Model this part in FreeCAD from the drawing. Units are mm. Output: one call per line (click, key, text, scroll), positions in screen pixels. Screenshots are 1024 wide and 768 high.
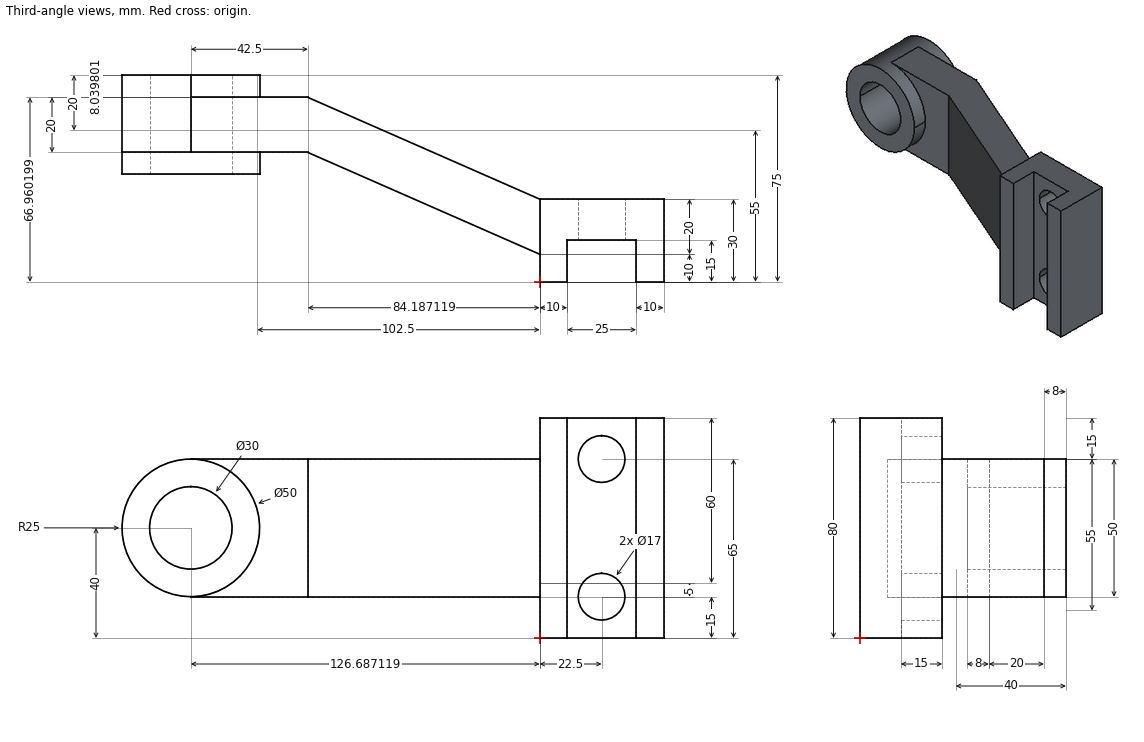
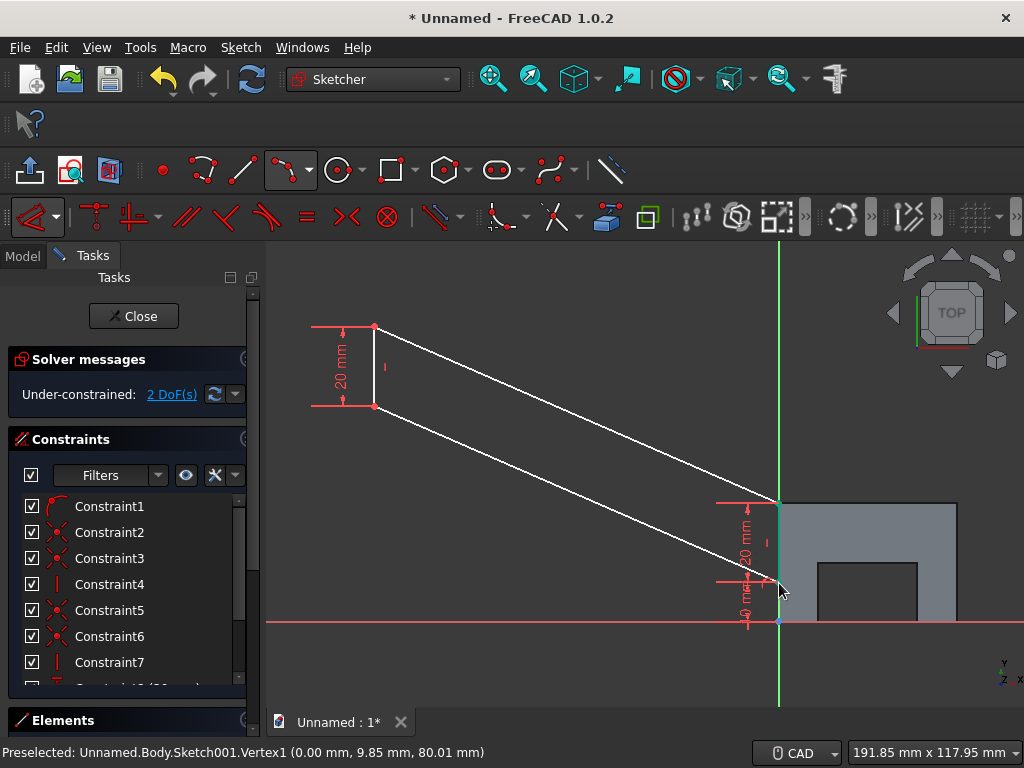
click(374, 327)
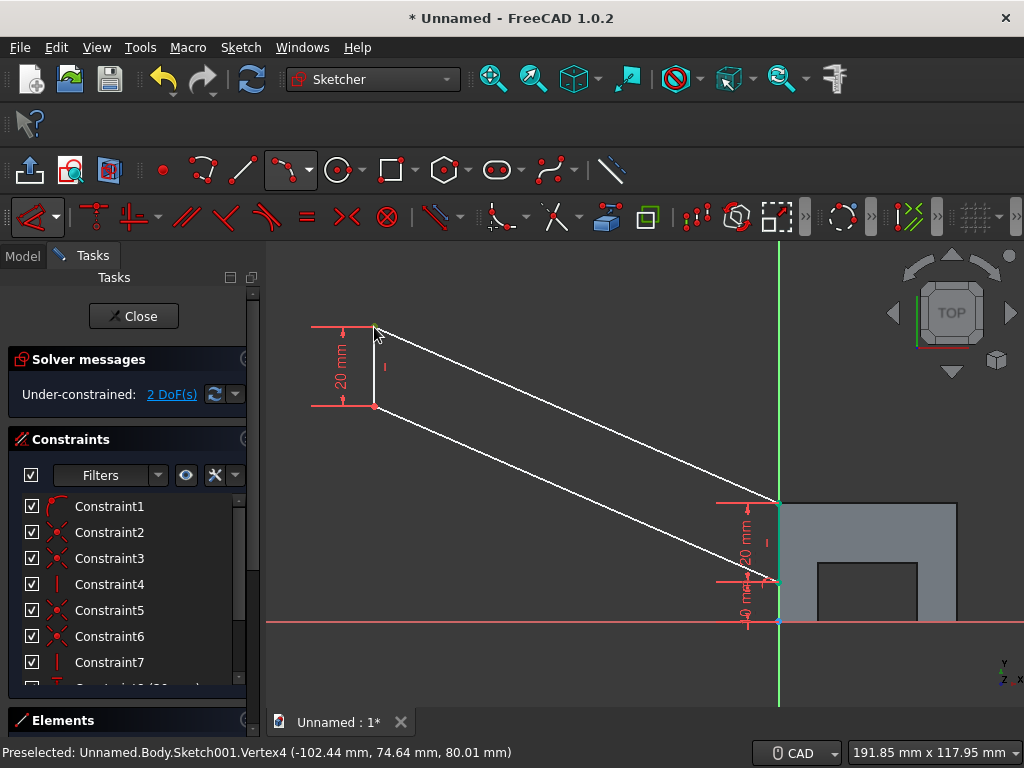
click(58, 218)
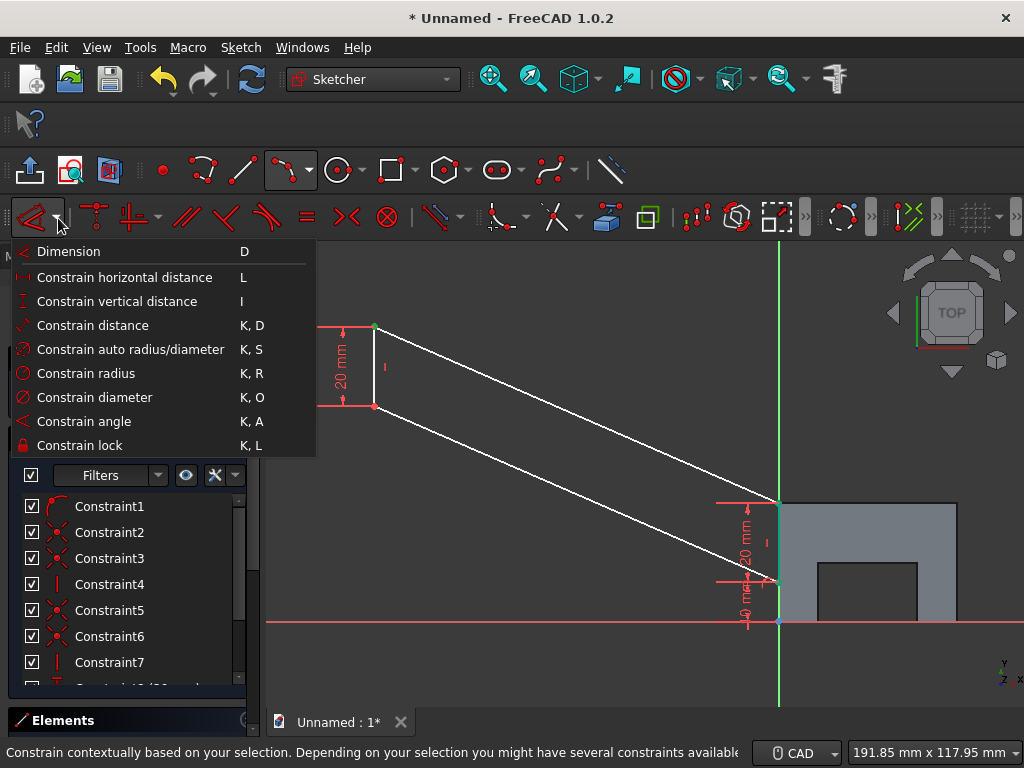
click(164, 301)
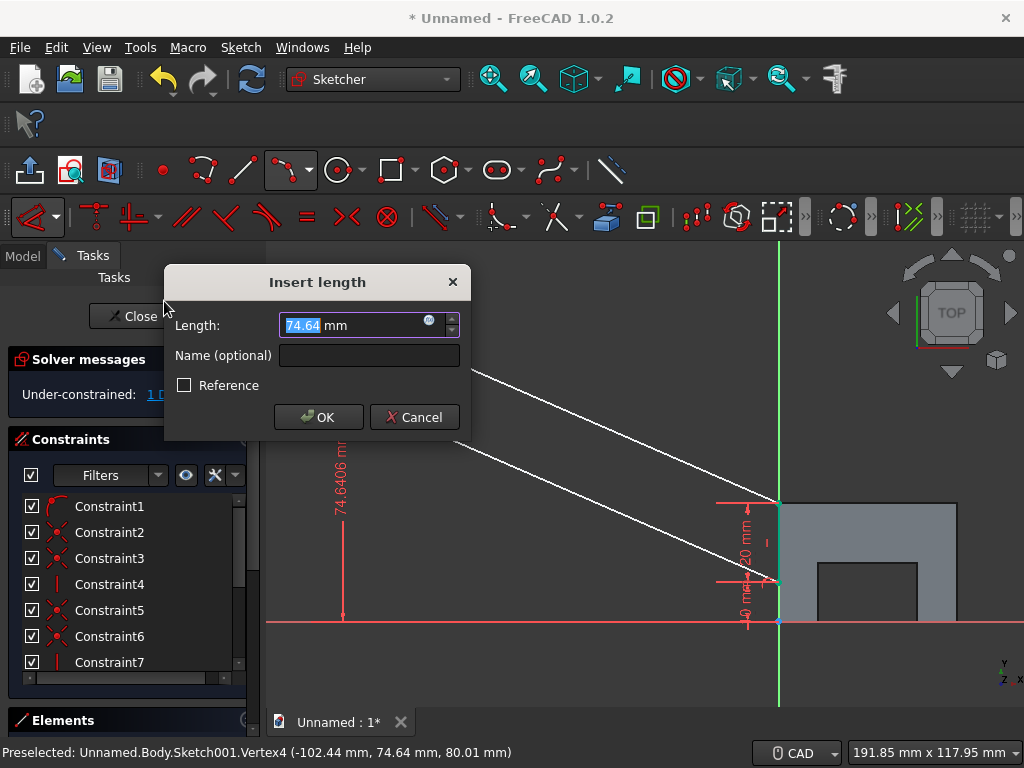
text(75)
key(Return)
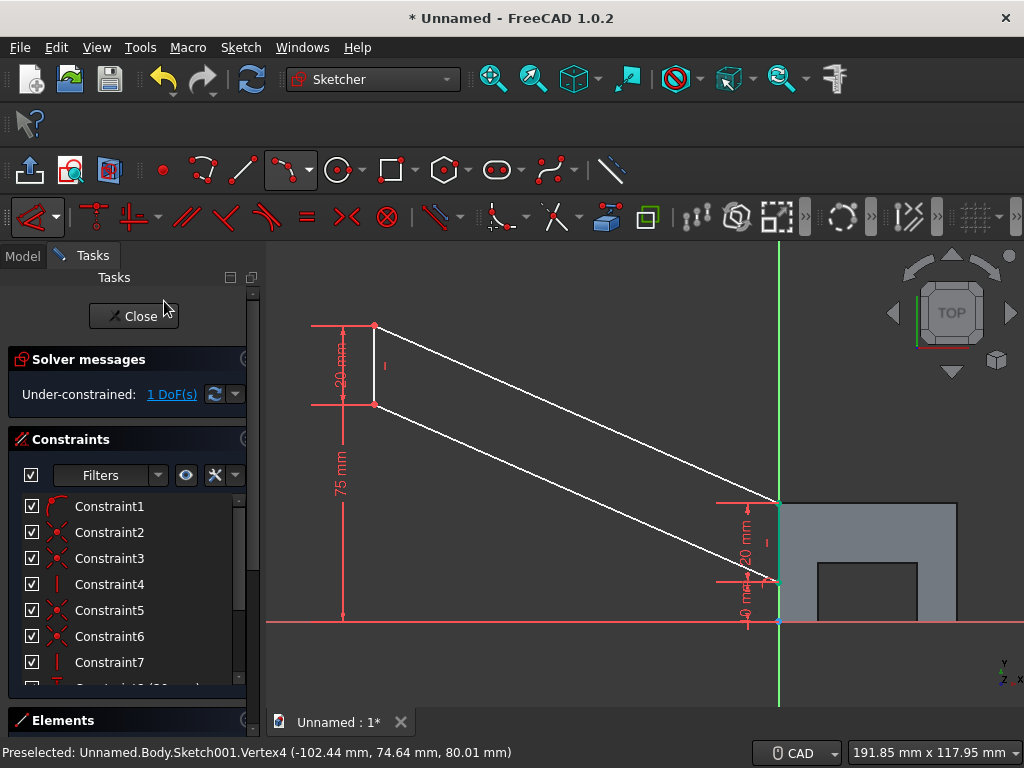
click(374, 326)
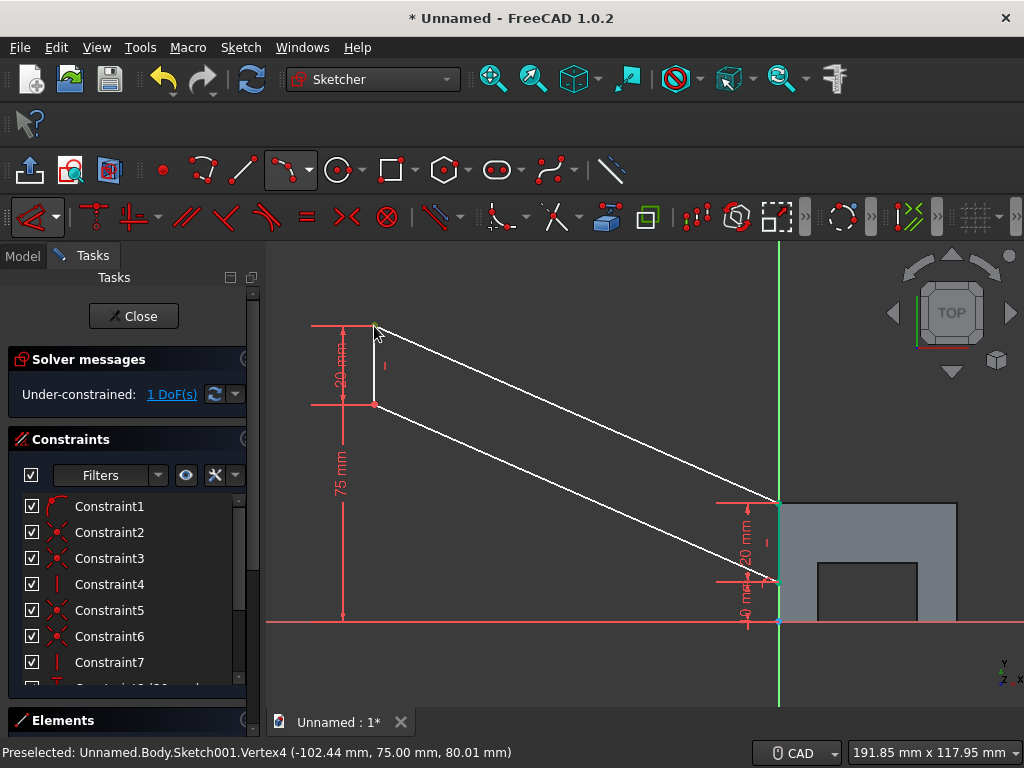
key(l)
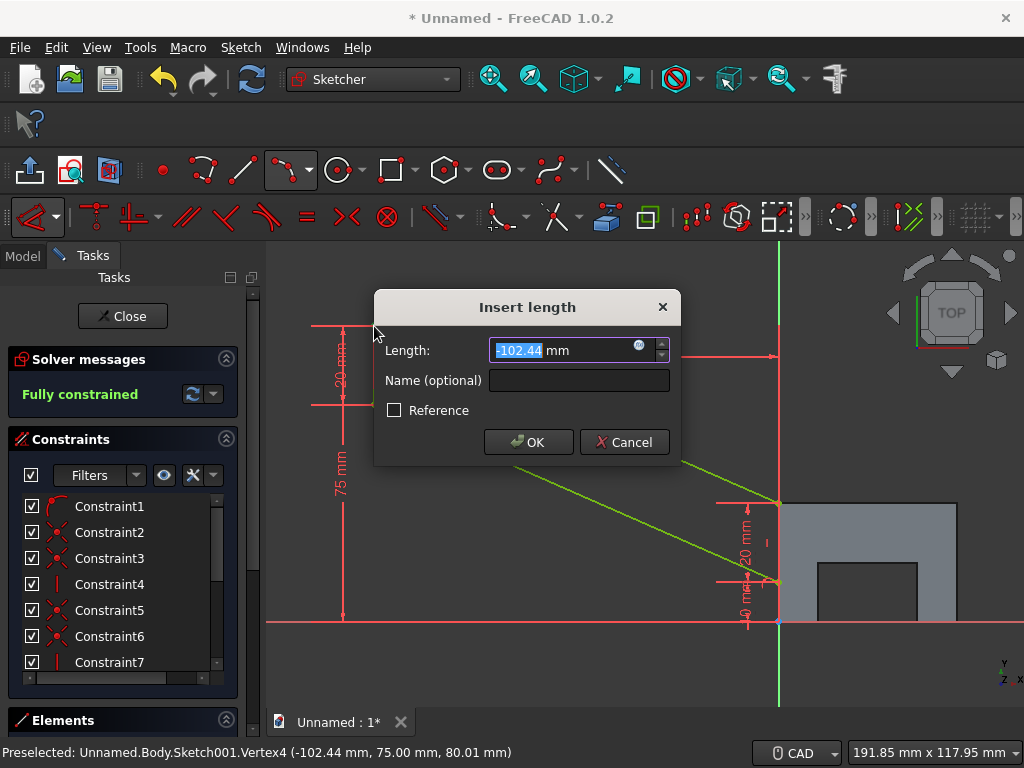
text(-102.5)
key(Return)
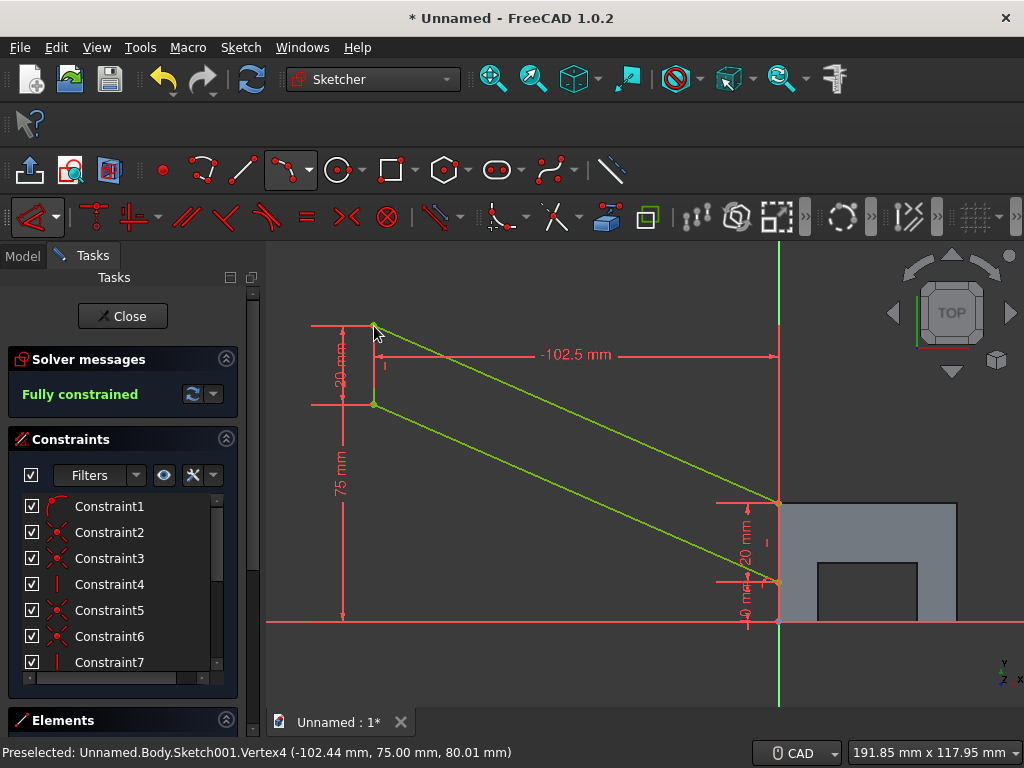
click(123, 316)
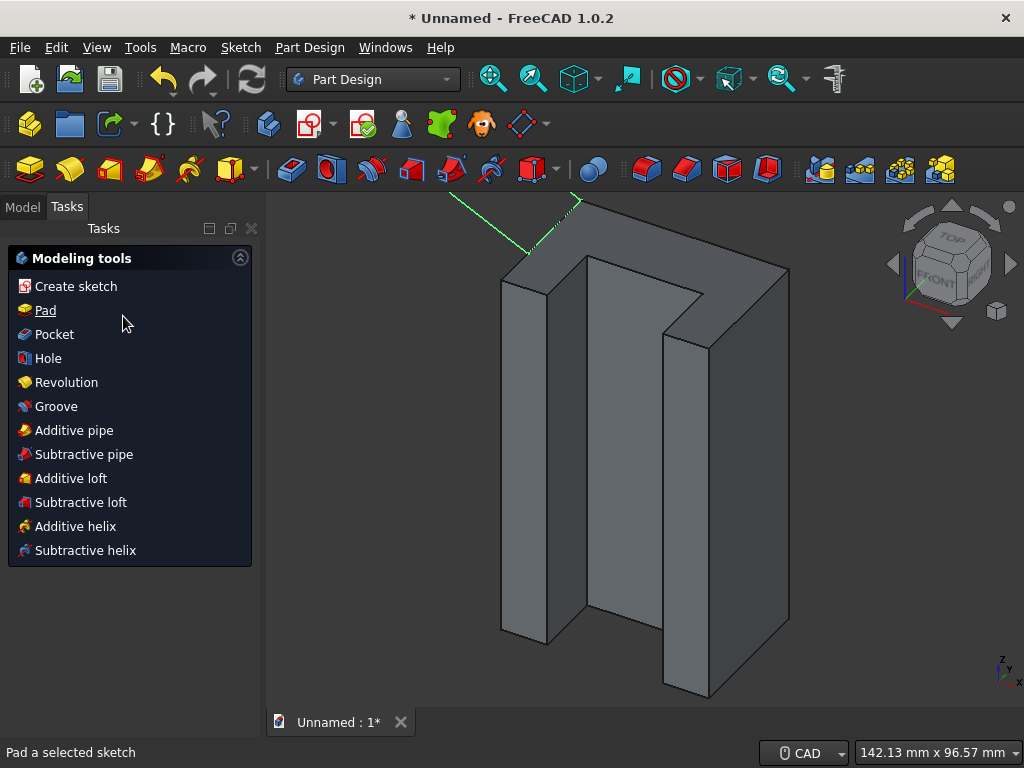
click(30, 170)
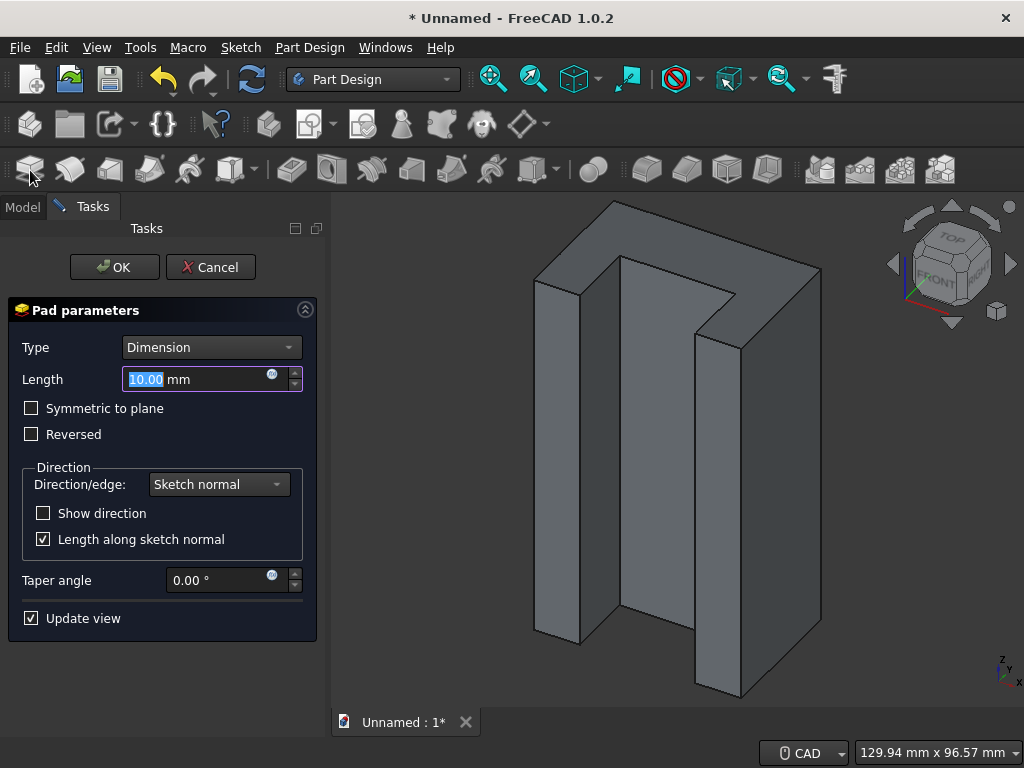
text(60)
key(Tab)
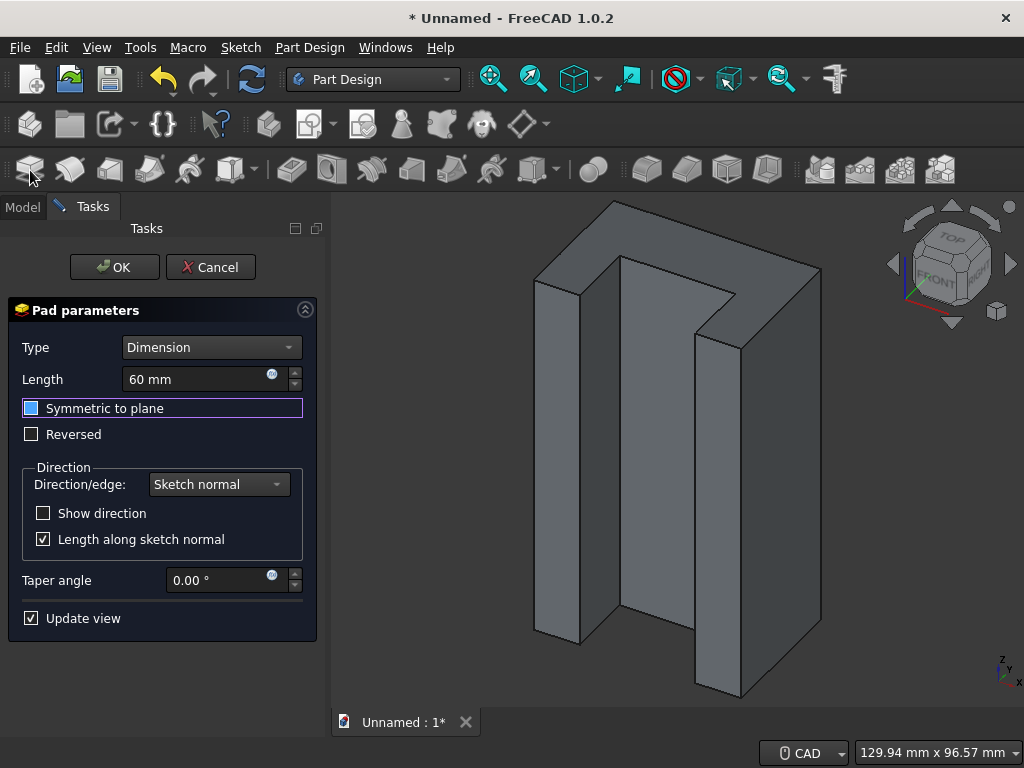
click(30, 434)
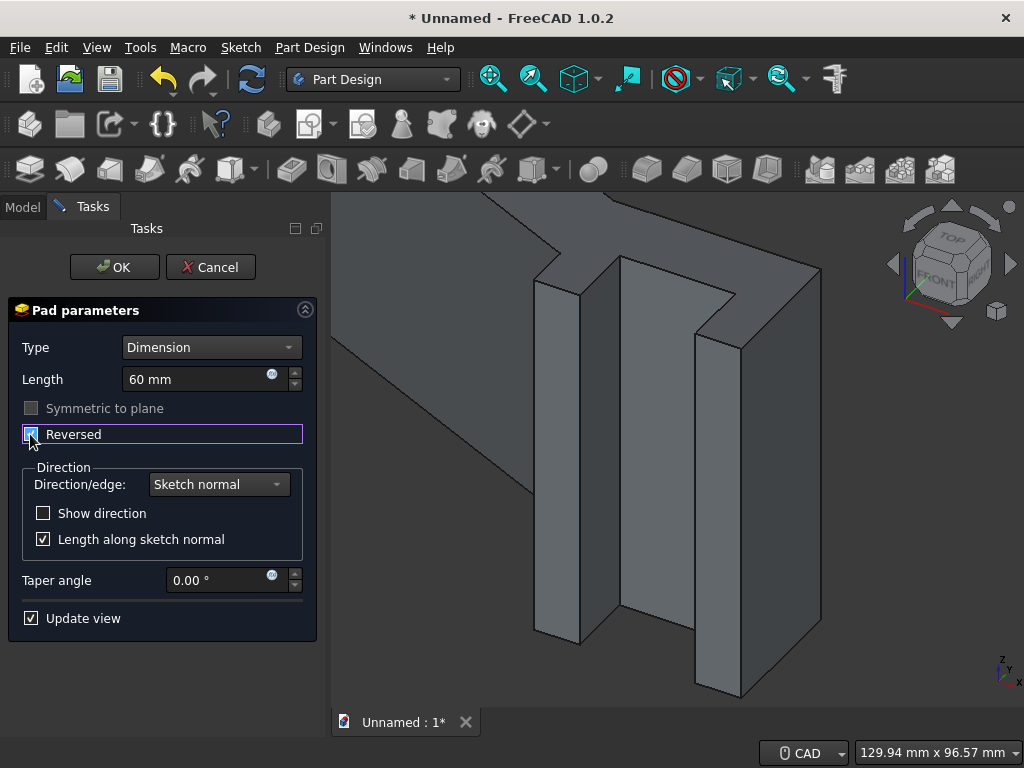
click(115, 267)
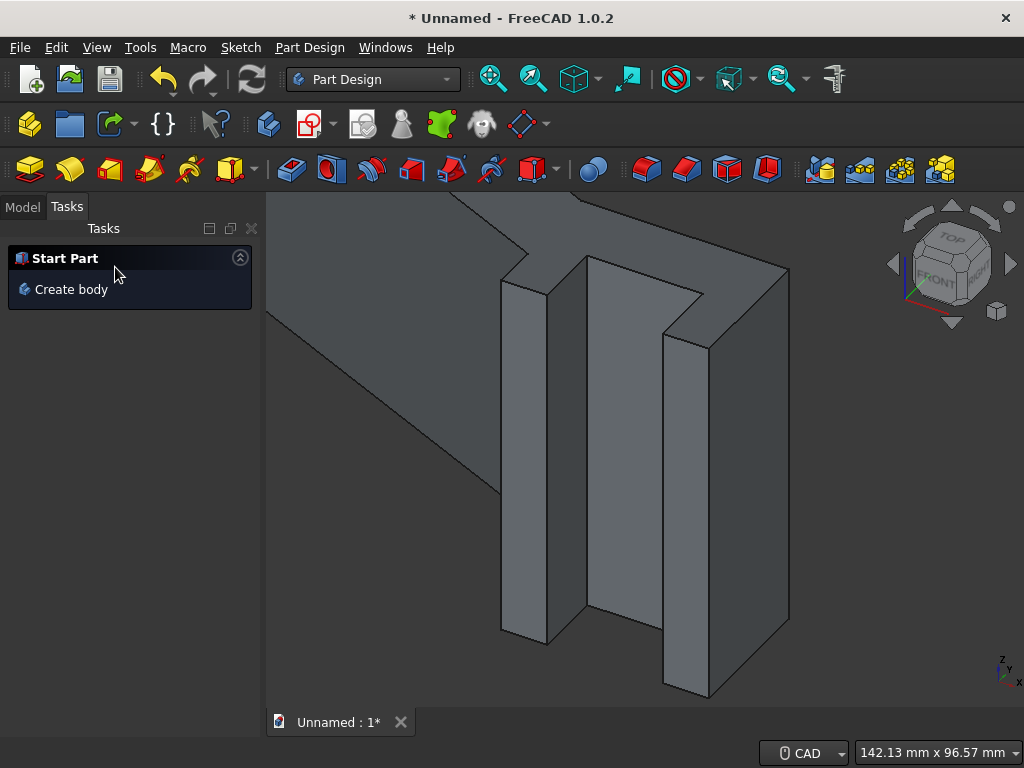
click(494, 80)